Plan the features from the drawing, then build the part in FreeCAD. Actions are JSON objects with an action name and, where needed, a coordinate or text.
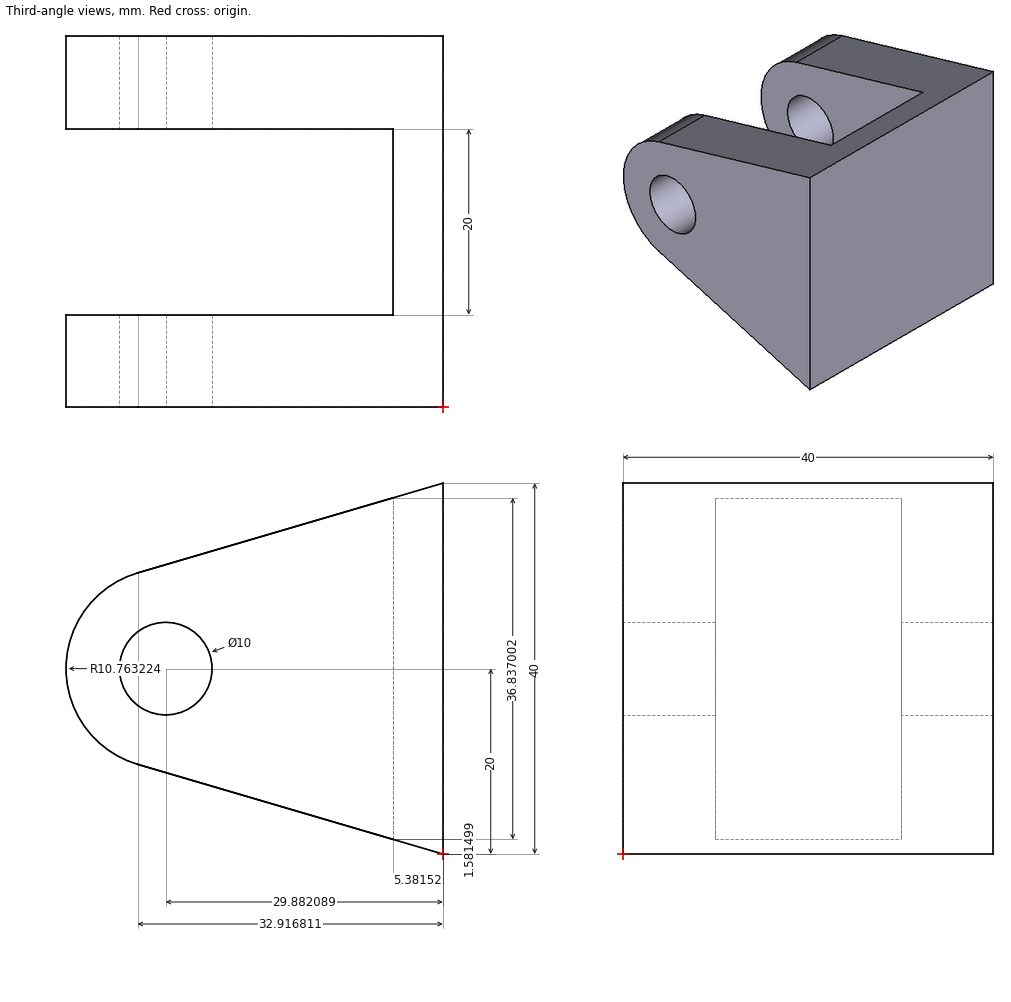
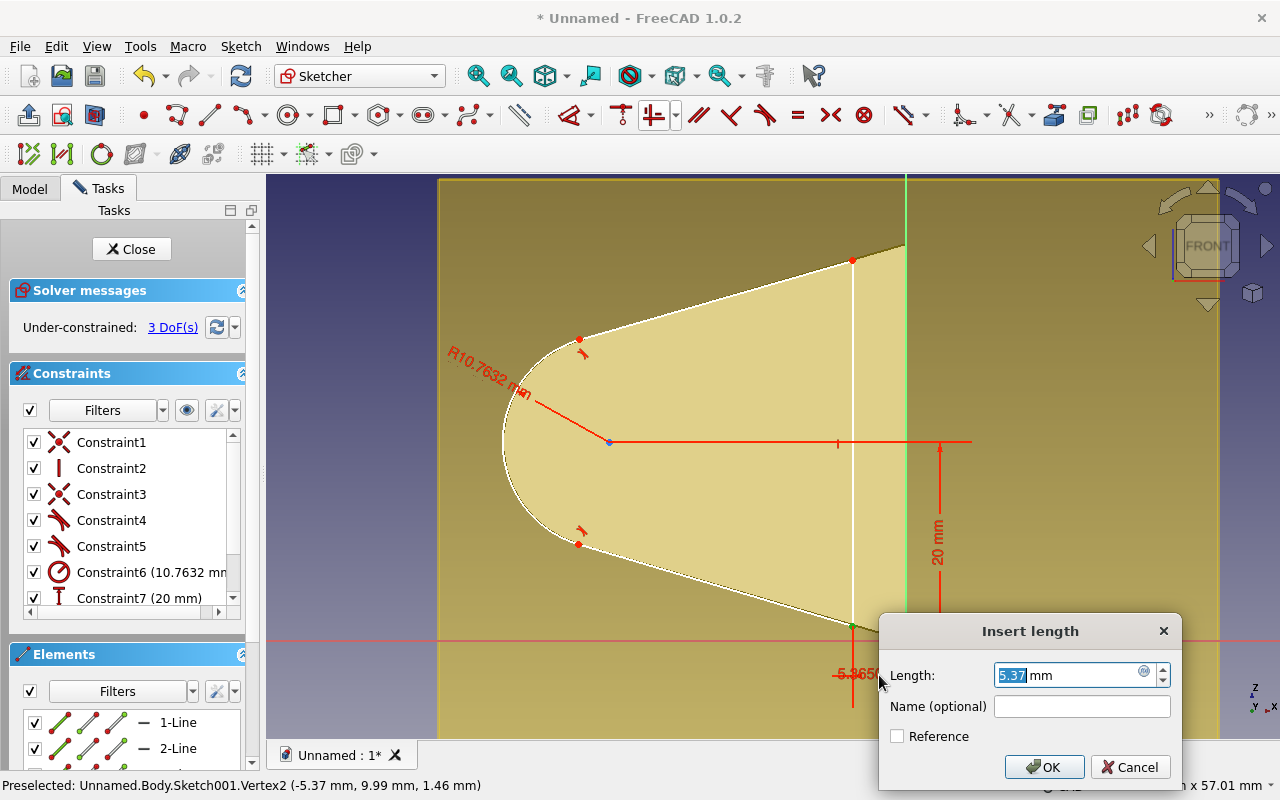
{"action": "type", "text": "5.38152"}
{"action": "key", "text": "Return"}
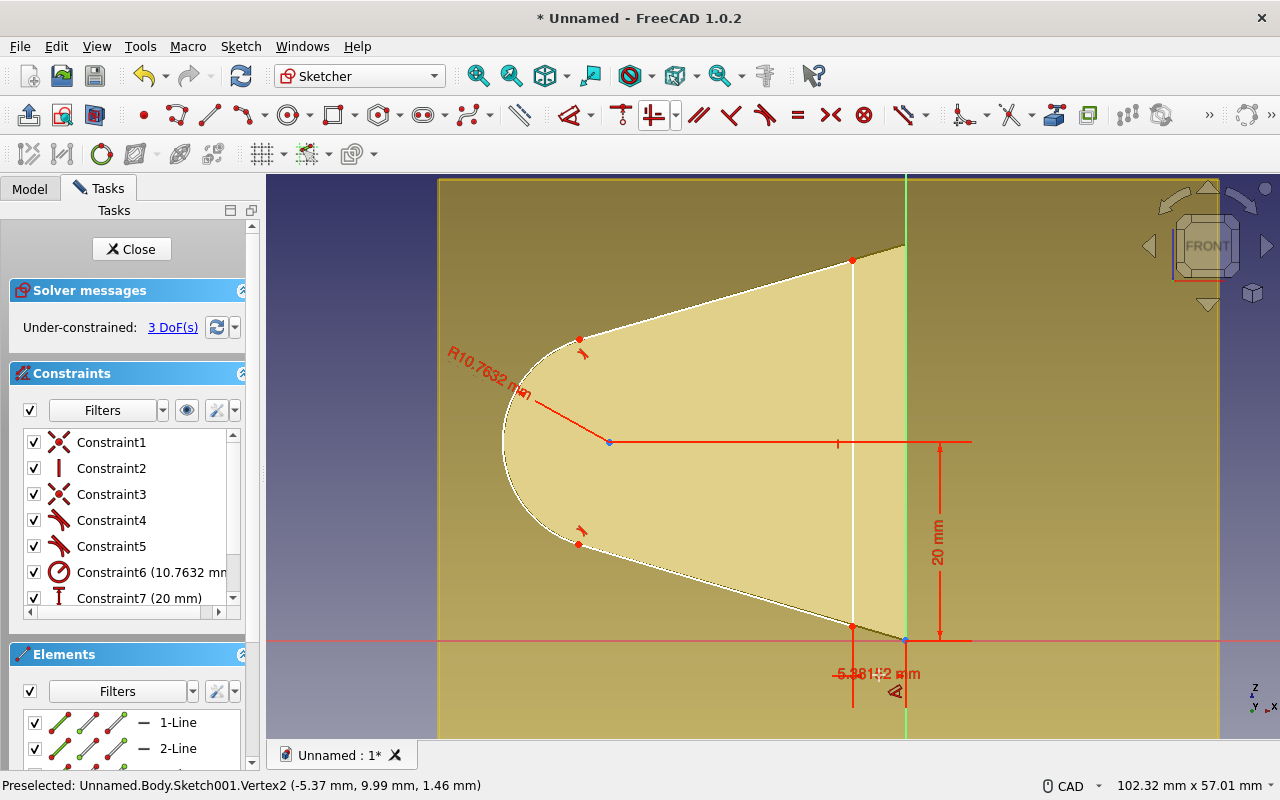
{"action": "left_click", "coordinate": [853, 517]}
{"action": "left_click", "coordinate": [887, 444]}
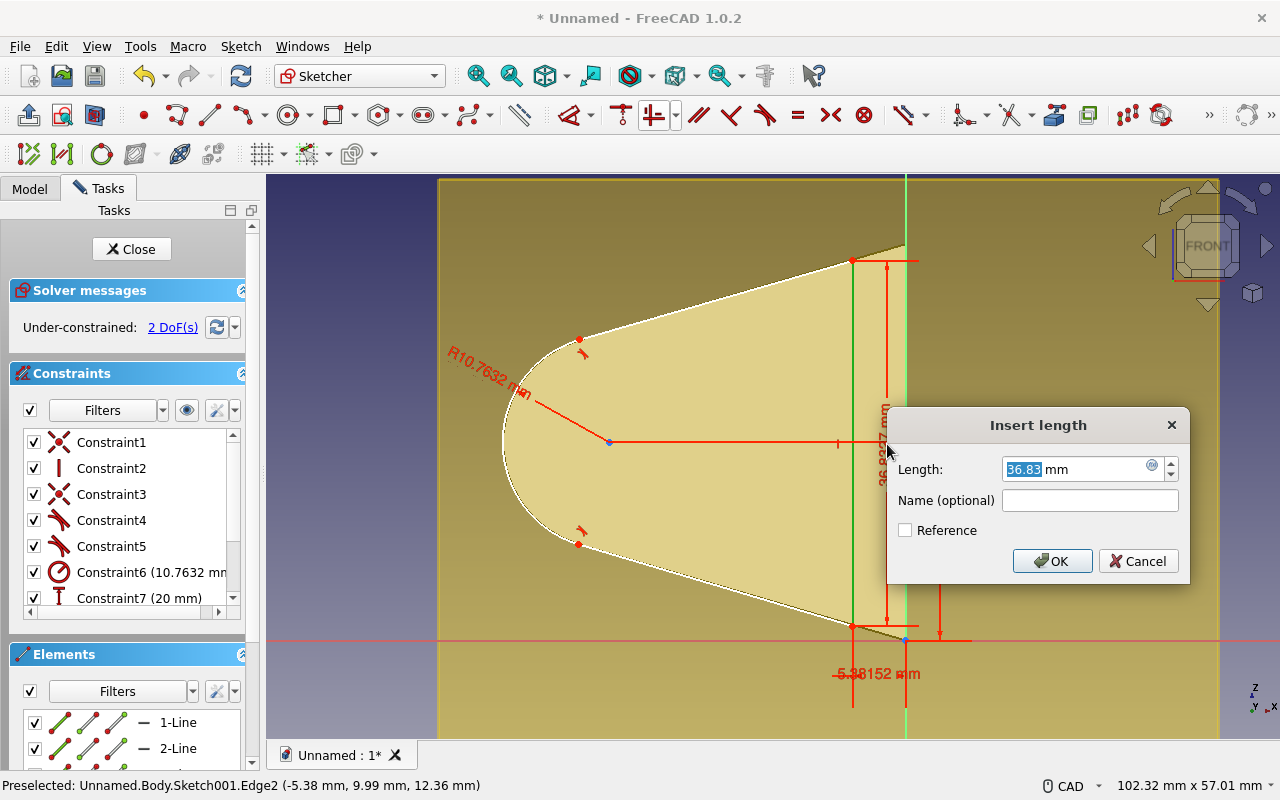
{"action": "type", "text": "36.837002"}
{"action": "key", "text": "Return"}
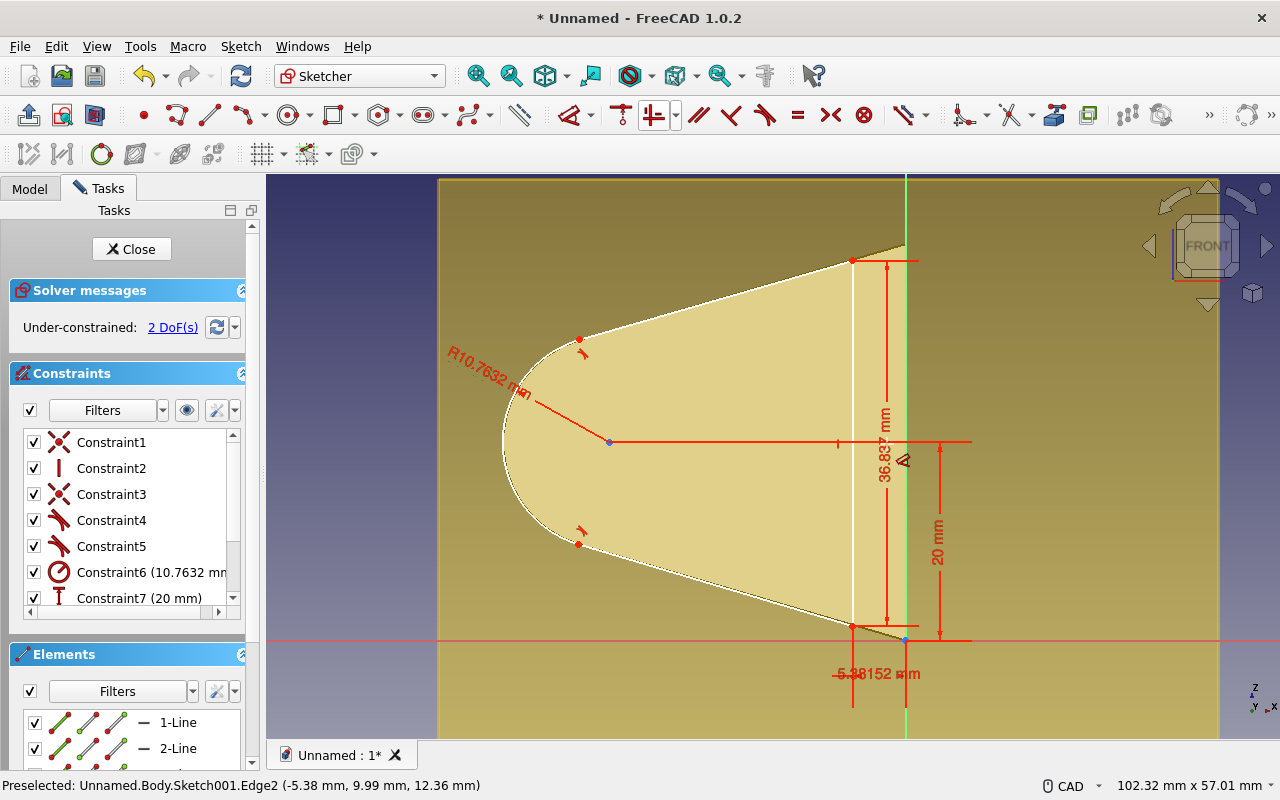
{"action": "scroll", "coordinate": [853, 626], "scroll_direction": "up", "scroll_amount": 5}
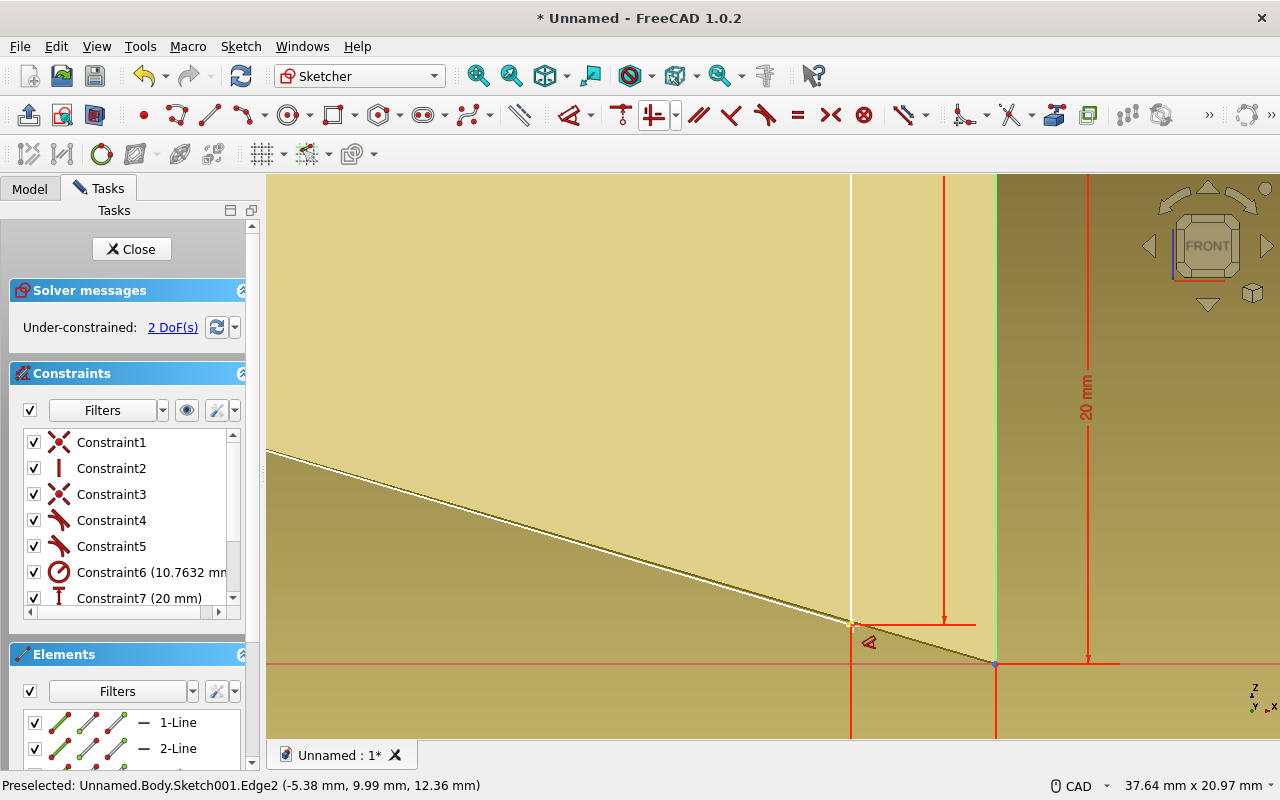
{"action": "left_click", "coordinate": [851, 625]}
{"action": "left_click", "coordinate": [1030, 644]}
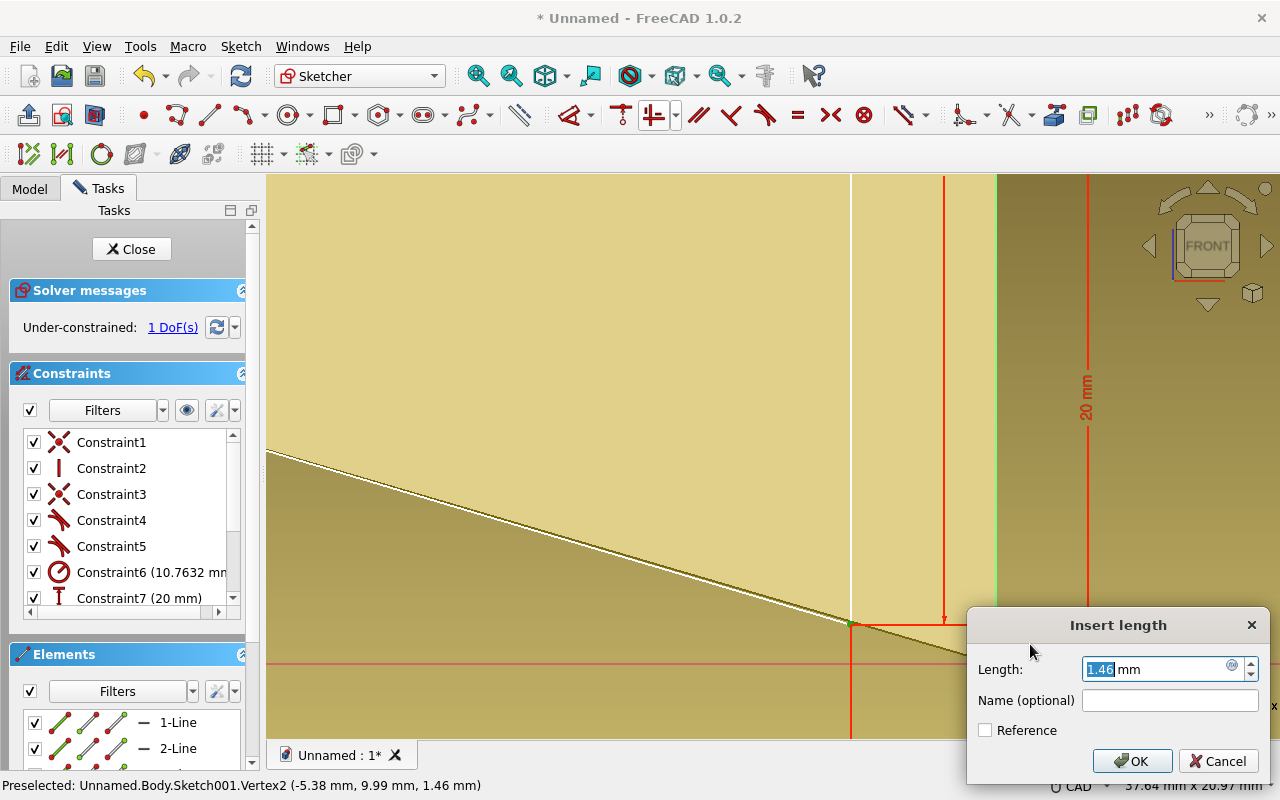
{"action": "type", "text": "1.581499"}
{"action": "key", "text": "Return"}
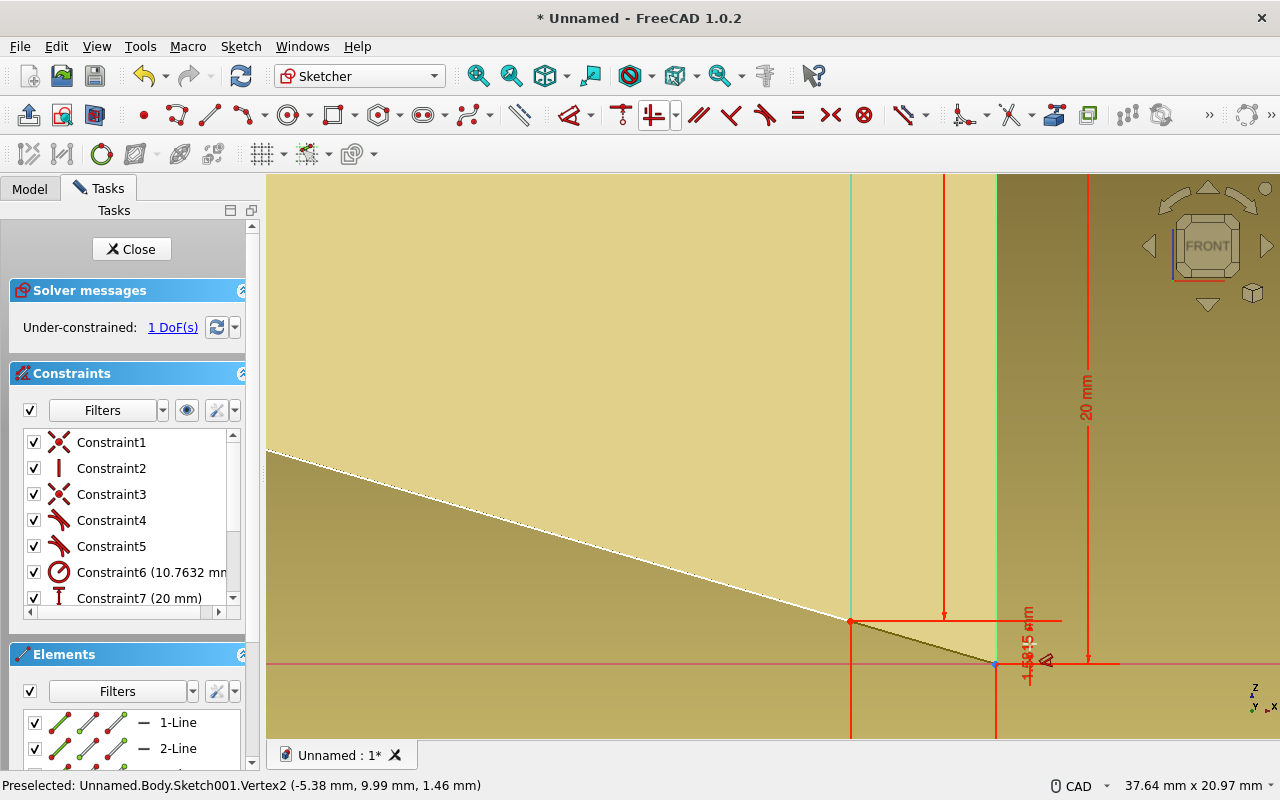
{"action": "scroll", "coordinate": [854, 637], "scroll_direction": "down", "scroll_amount": 5}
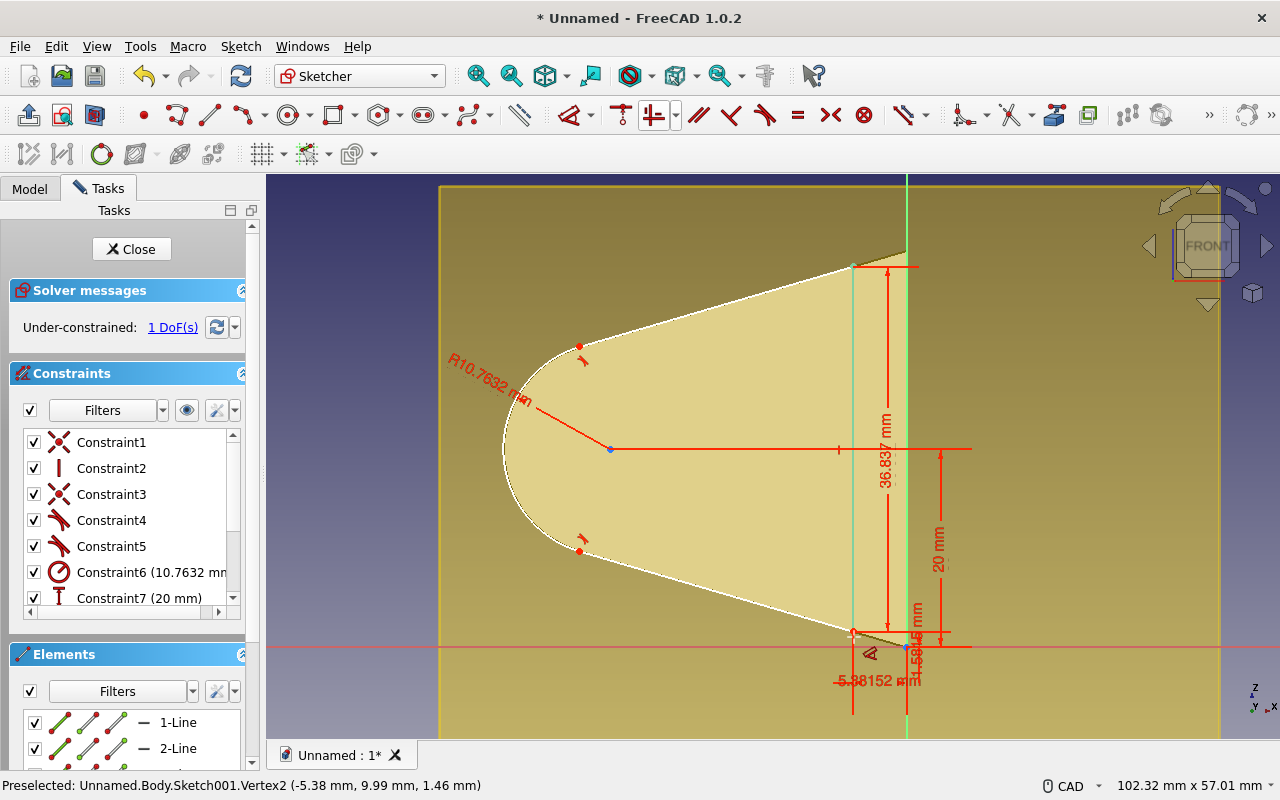
{"action": "left_click", "coordinate": [580, 552]}
{"action": "left_click", "coordinate": [743, 681]}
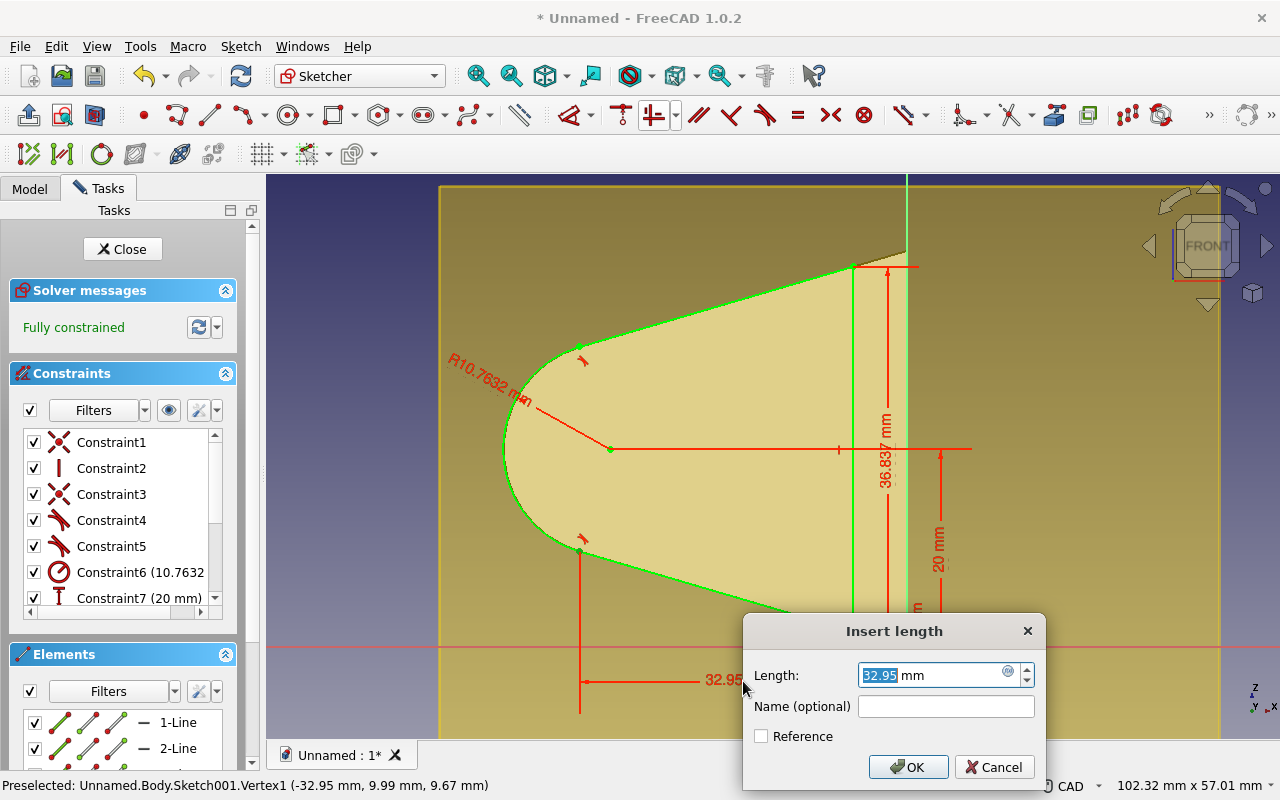
{"action": "type", "text": "32.916811"}
{"action": "key", "text": "Return"}
{"action": "key", "text": "Escape"}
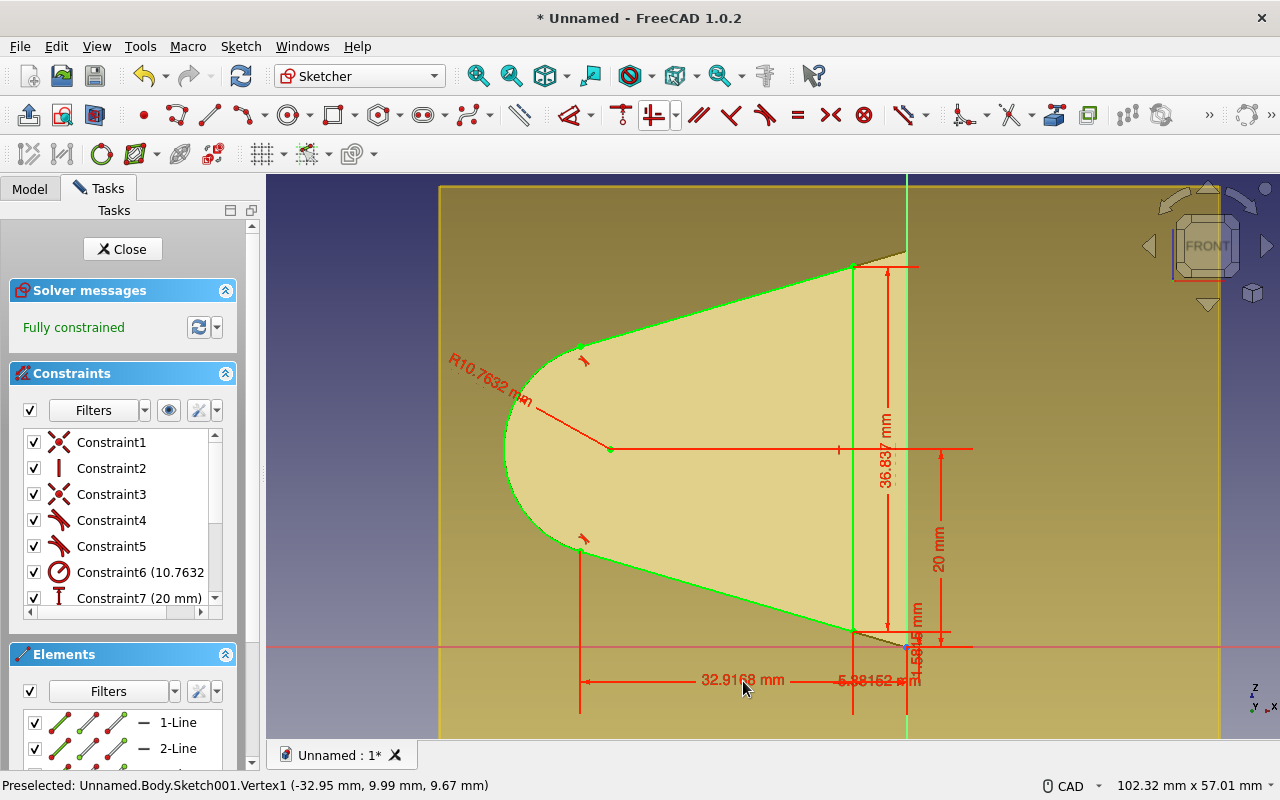
{"action": "left_click", "coordinate": [123, 249]}